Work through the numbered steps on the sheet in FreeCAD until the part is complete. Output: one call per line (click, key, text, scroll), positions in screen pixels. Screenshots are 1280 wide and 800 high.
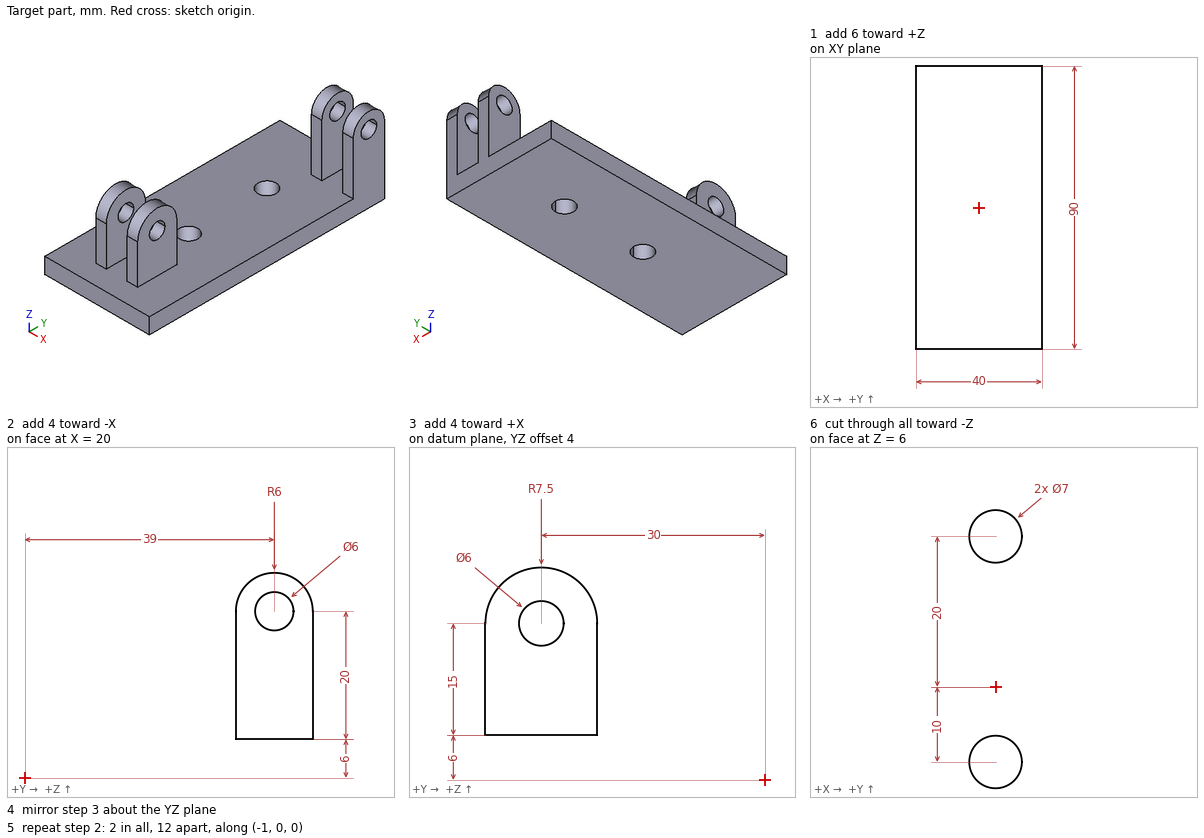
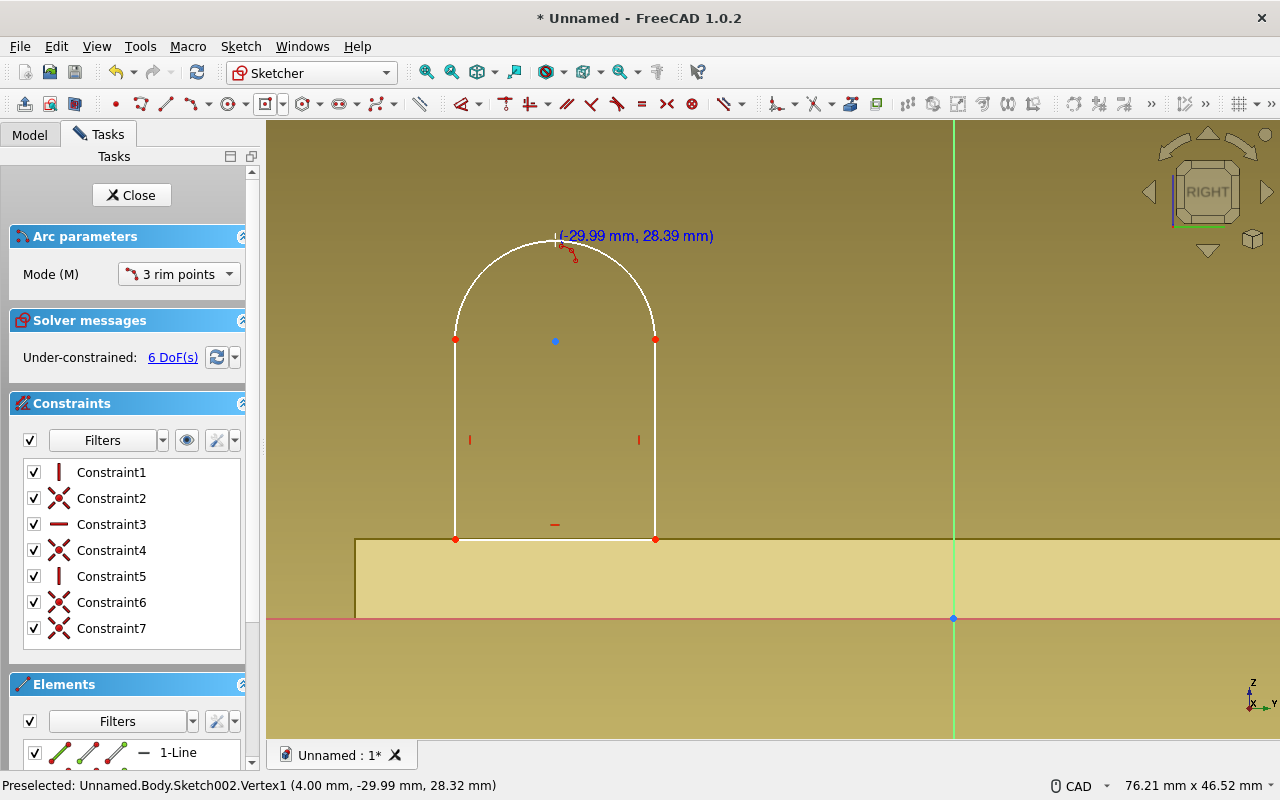
click(228, 104)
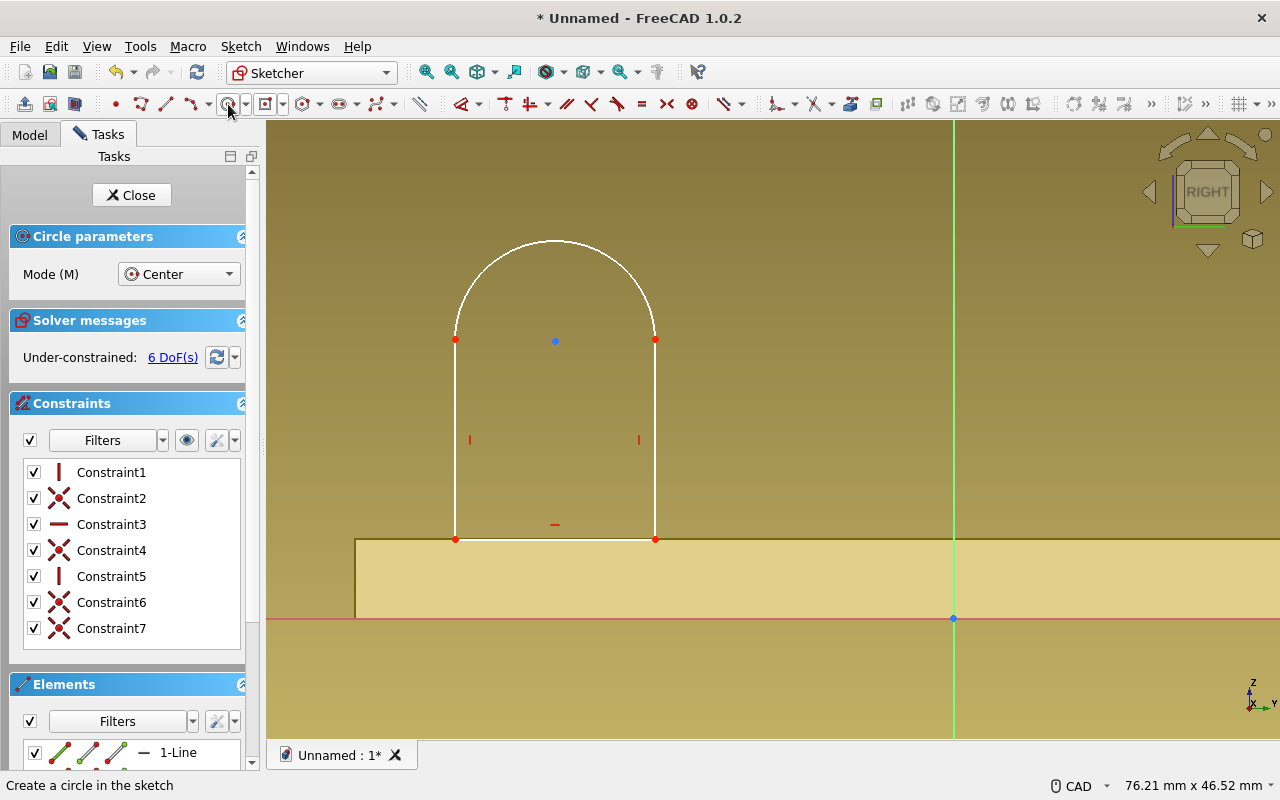
click(555, 339)
move(583, 311)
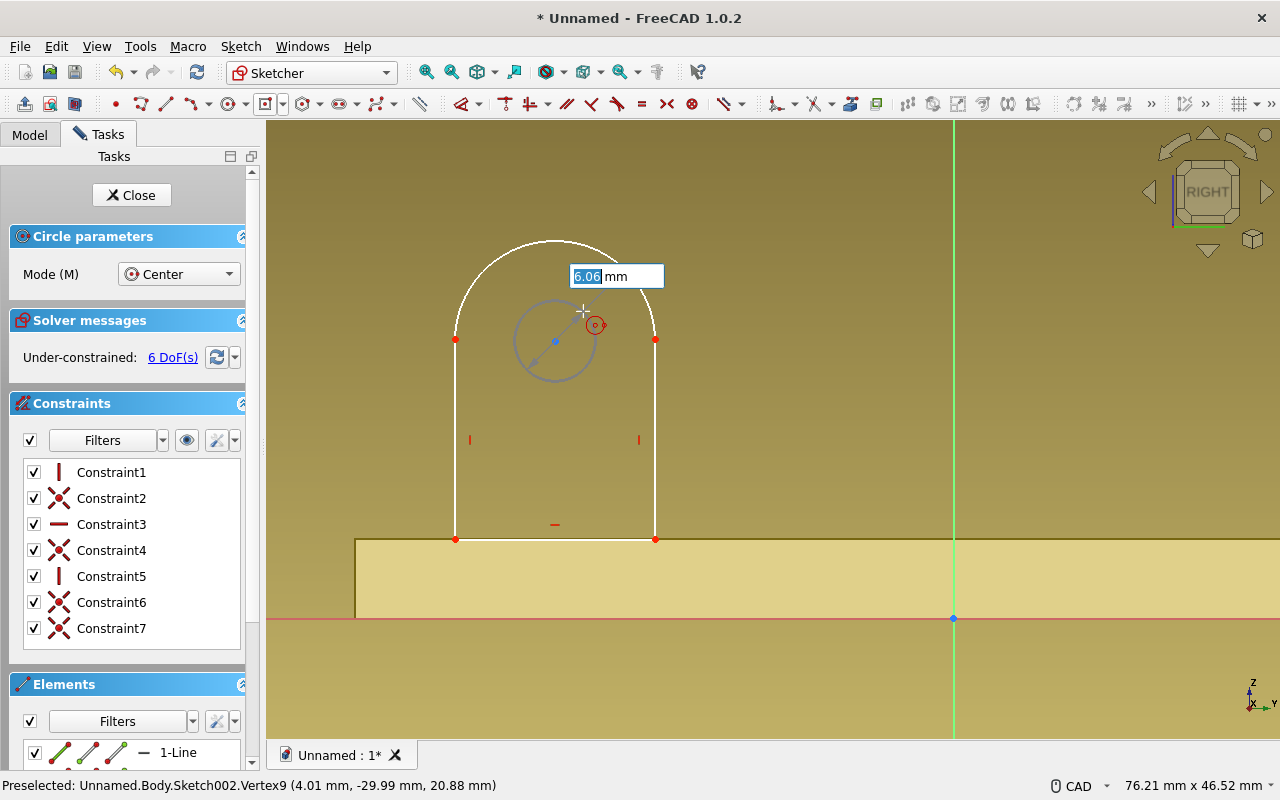
text(6)
key(Return)
key(Escape)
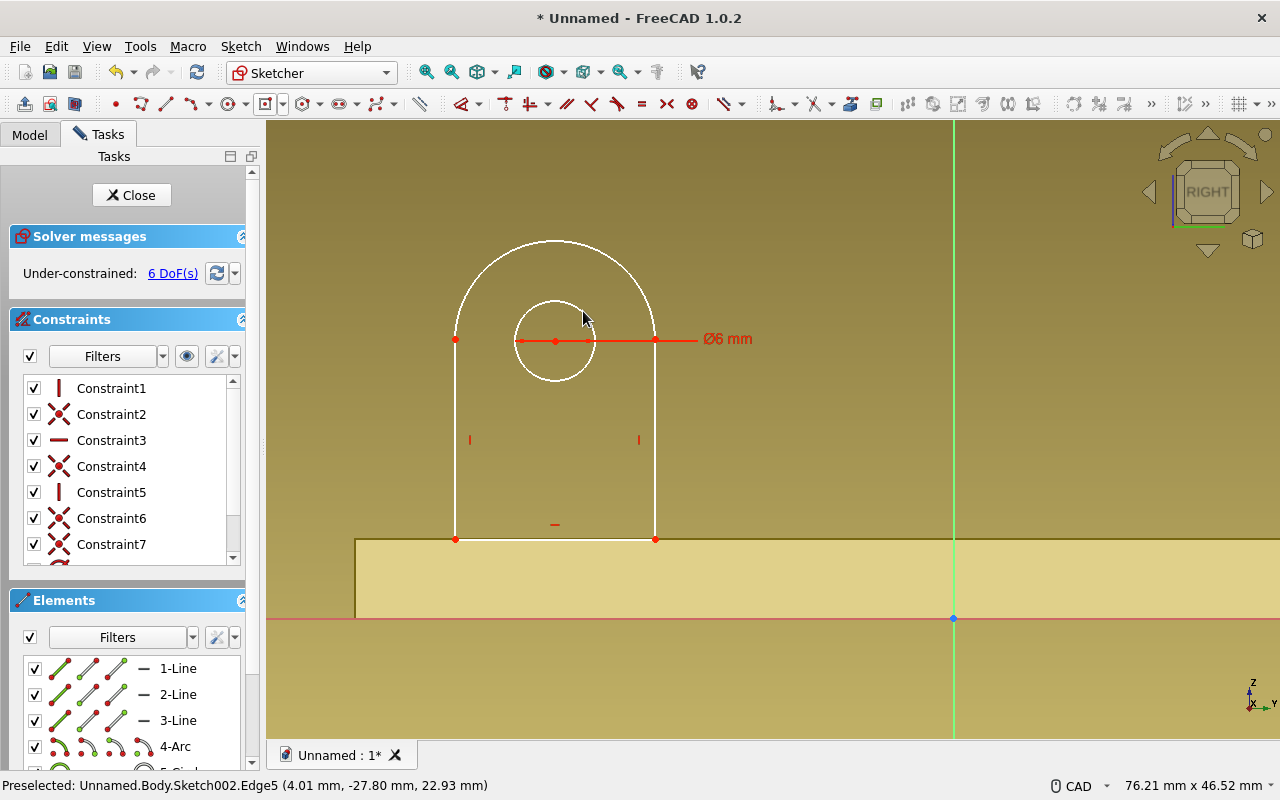
click(455, 400)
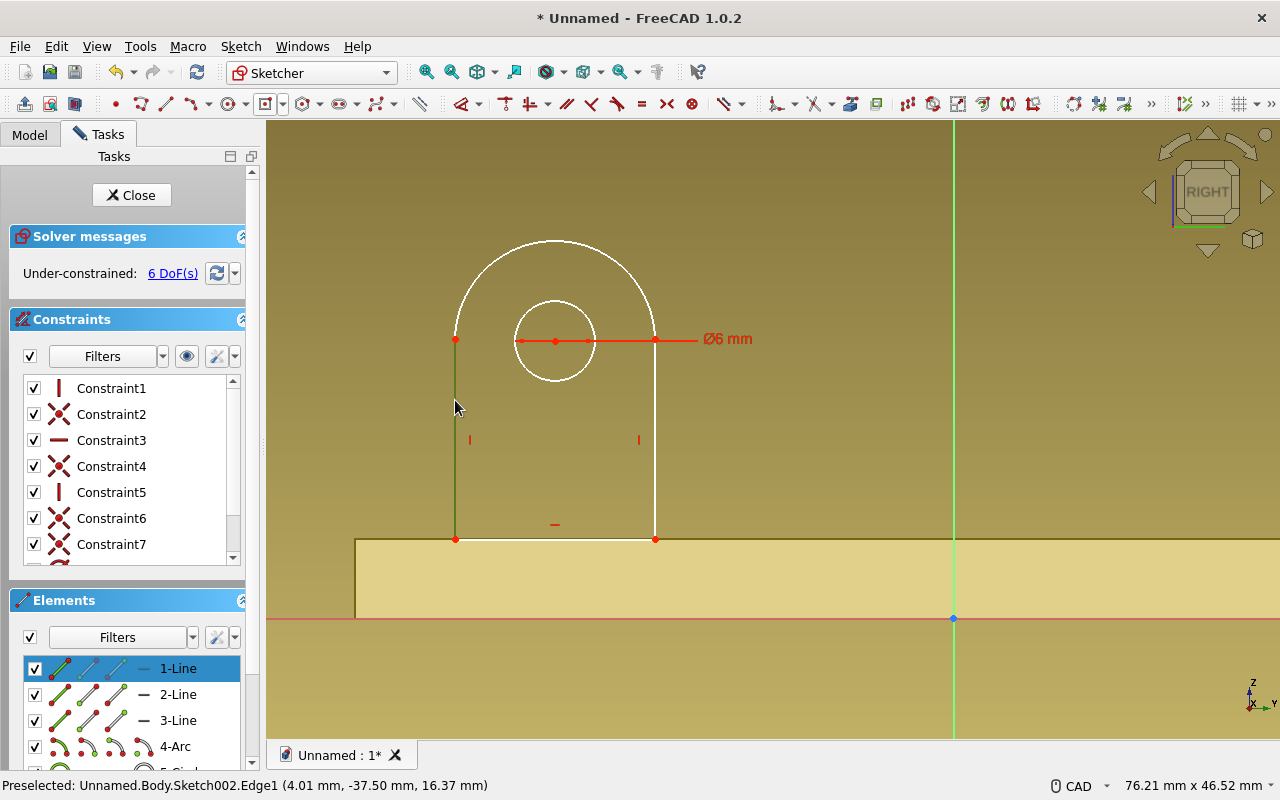
click(613, 260)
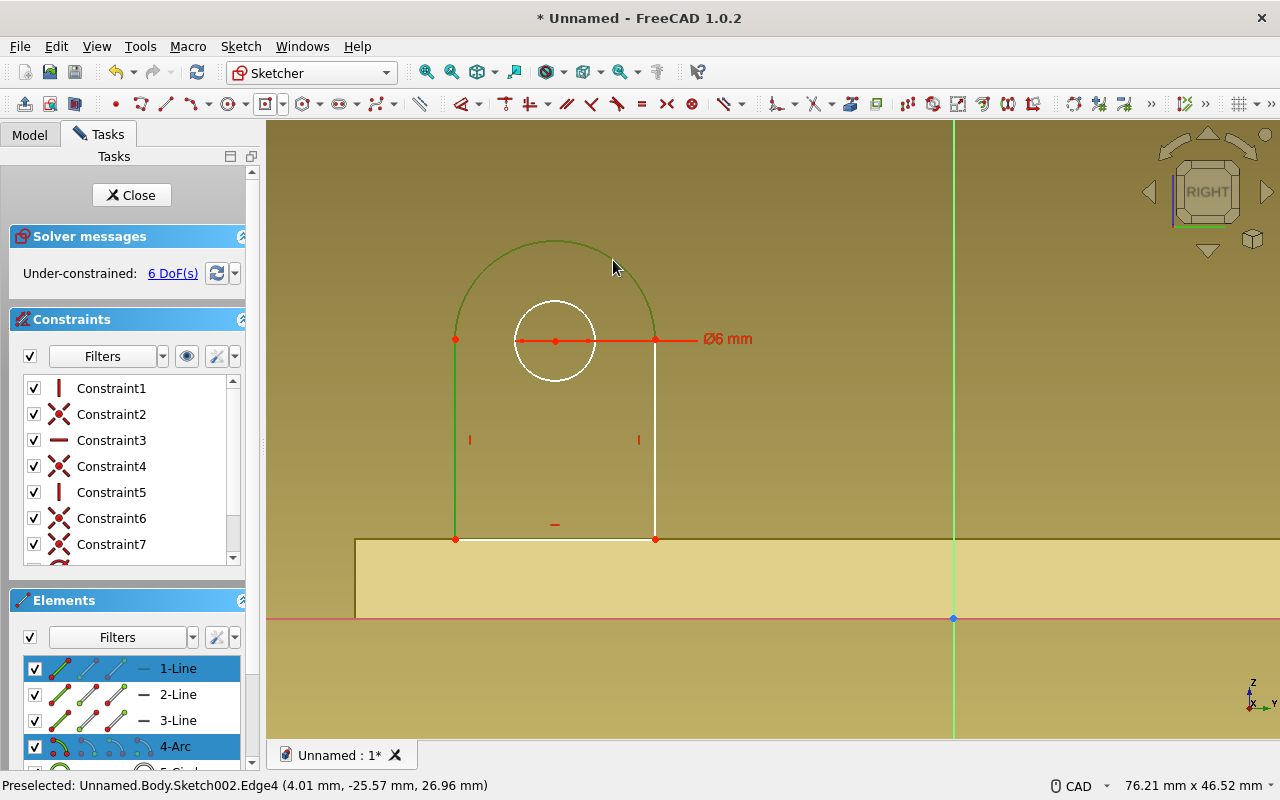
click(617, 104)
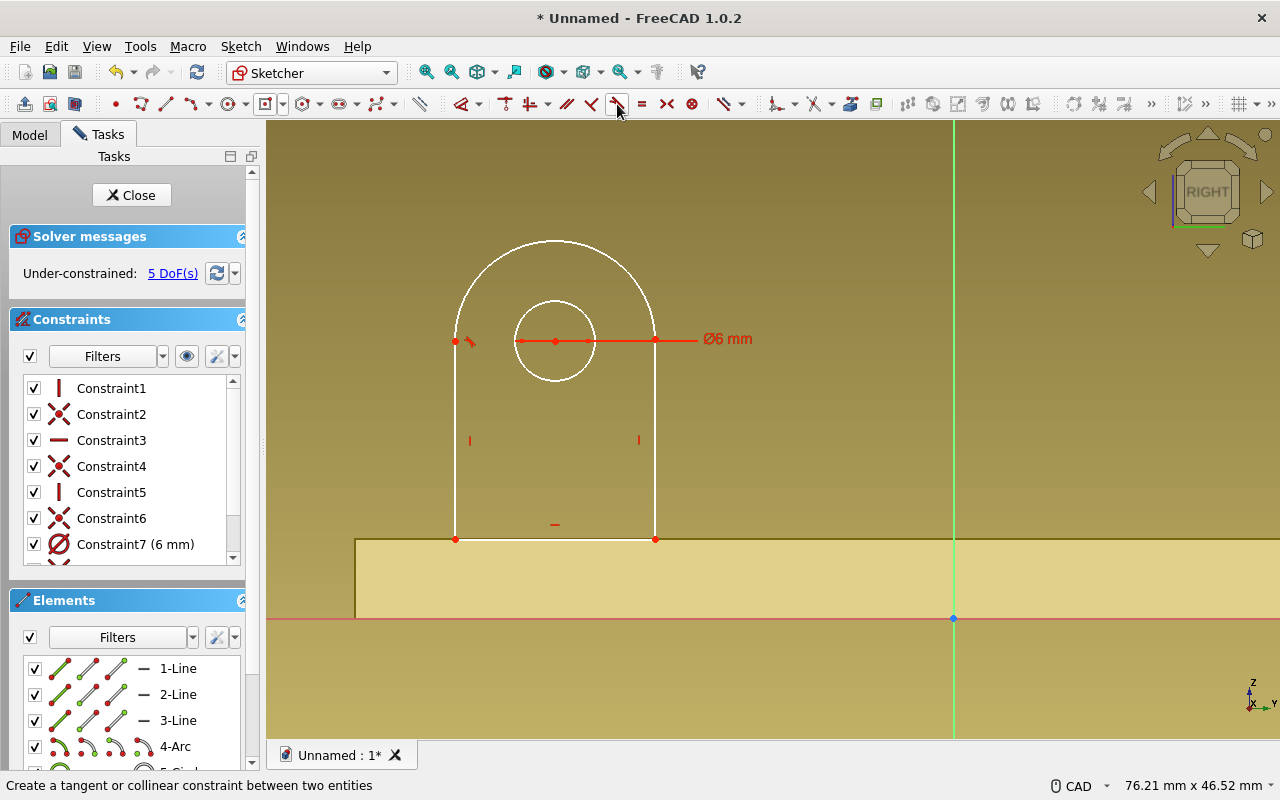
click(655, 480)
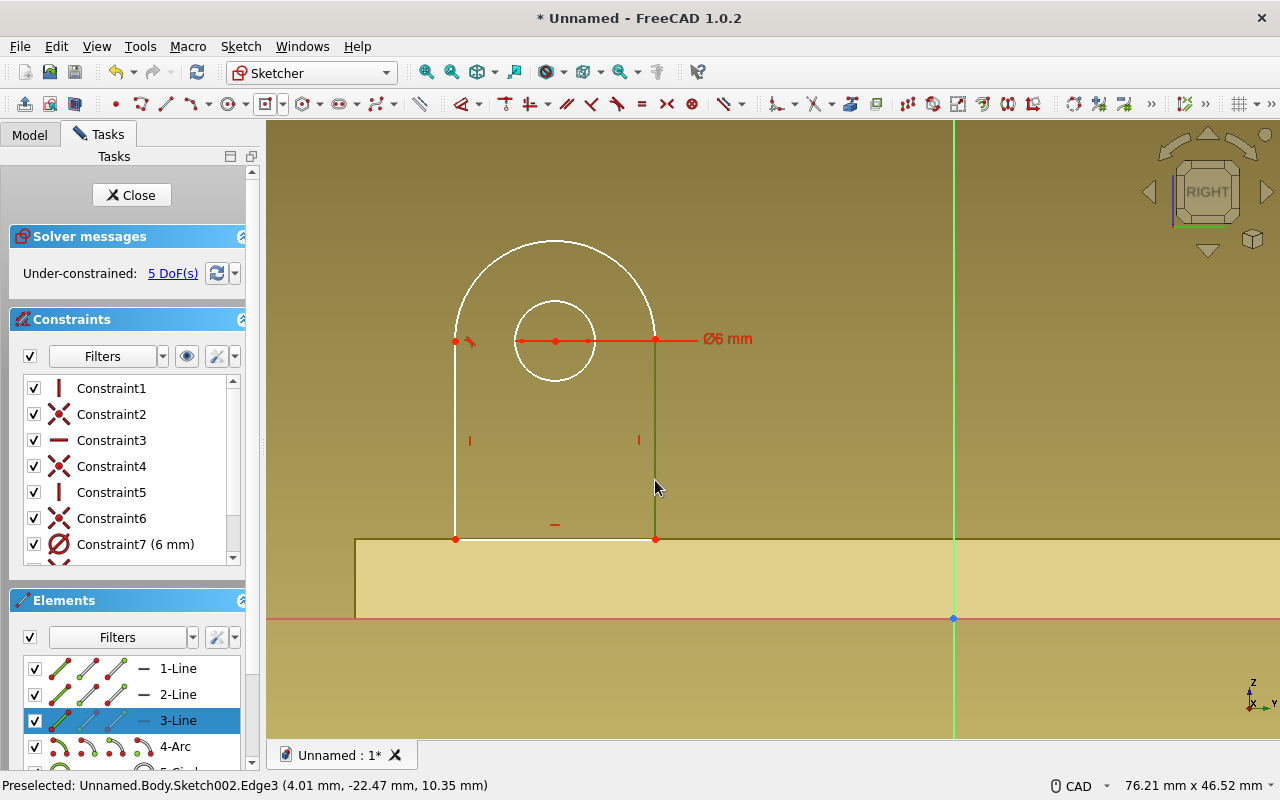
click(613, 260)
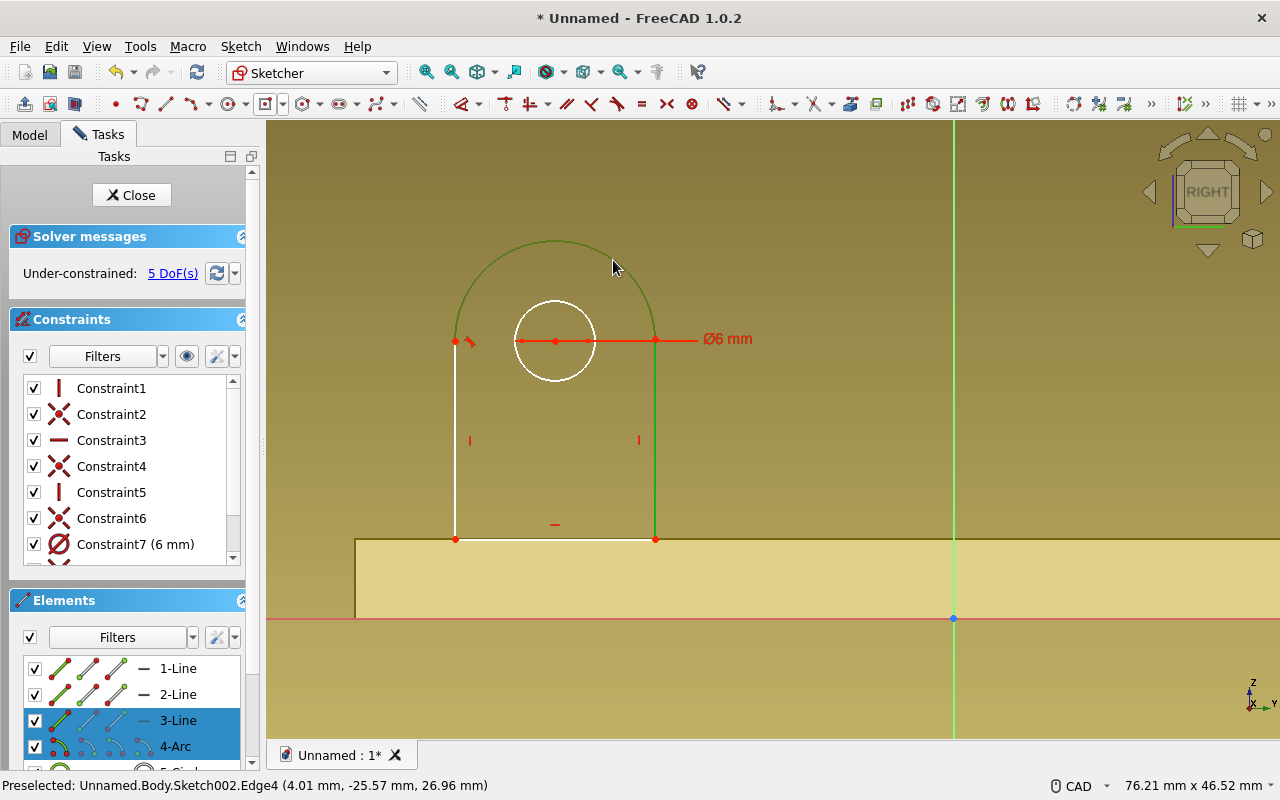
click(617, 104)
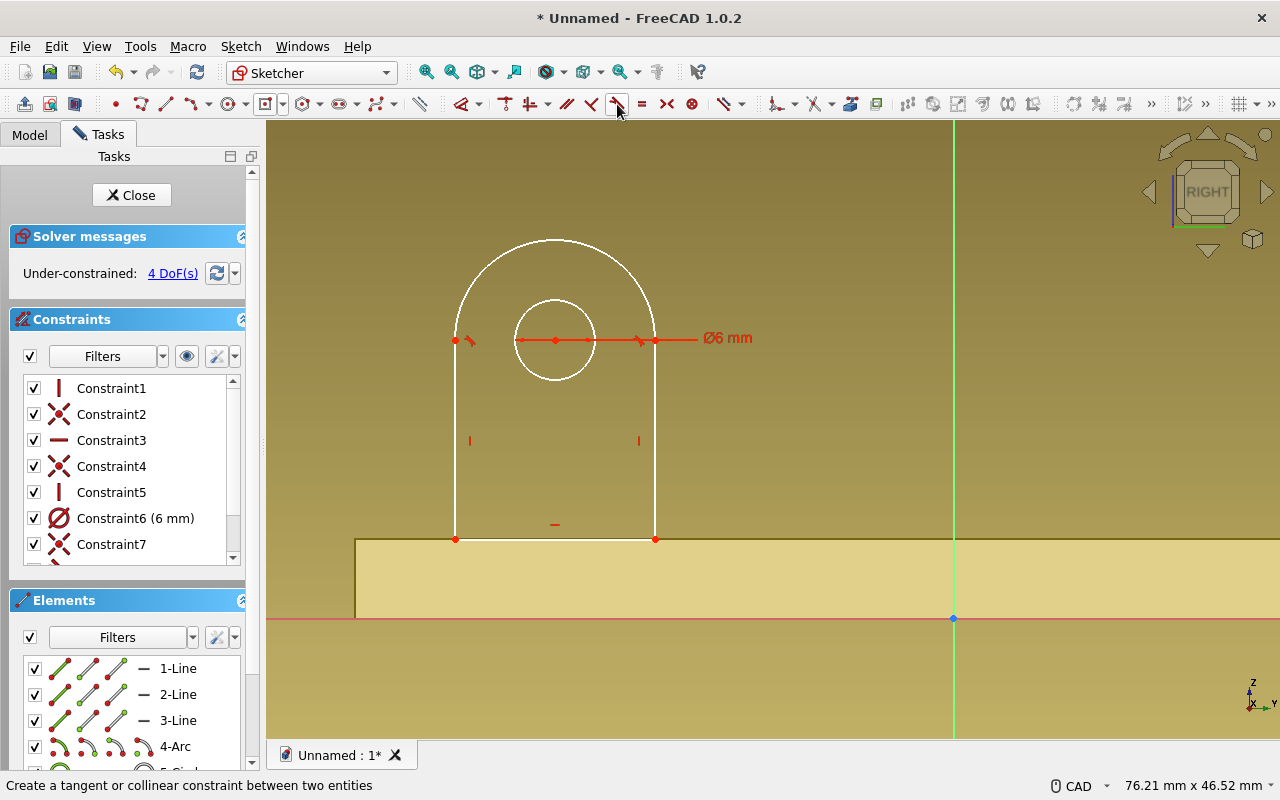
click(460, 104)